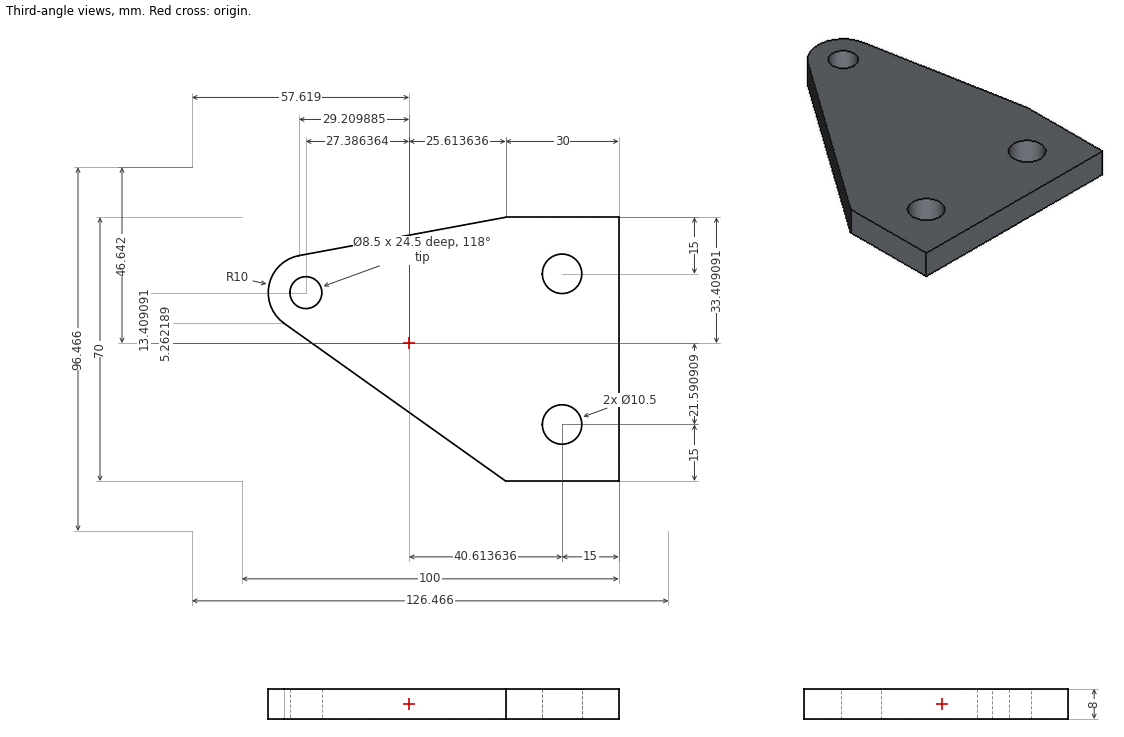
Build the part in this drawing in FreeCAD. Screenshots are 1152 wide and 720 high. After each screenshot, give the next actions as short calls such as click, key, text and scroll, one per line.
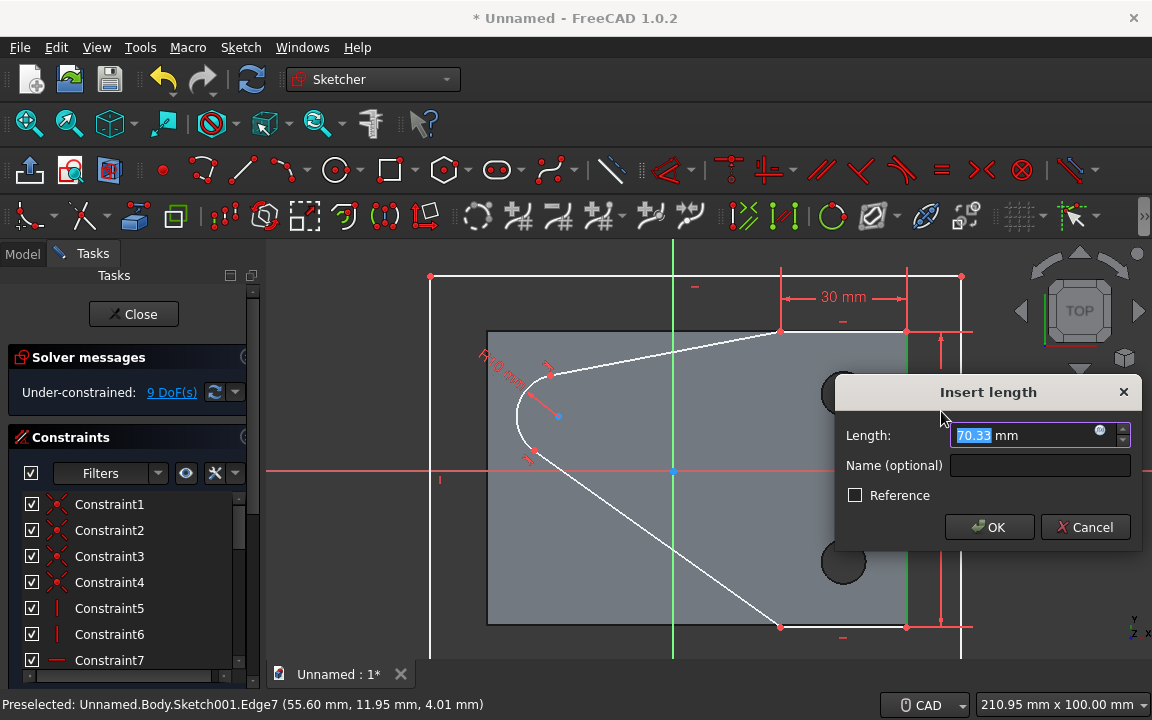
text(70)
key(Return)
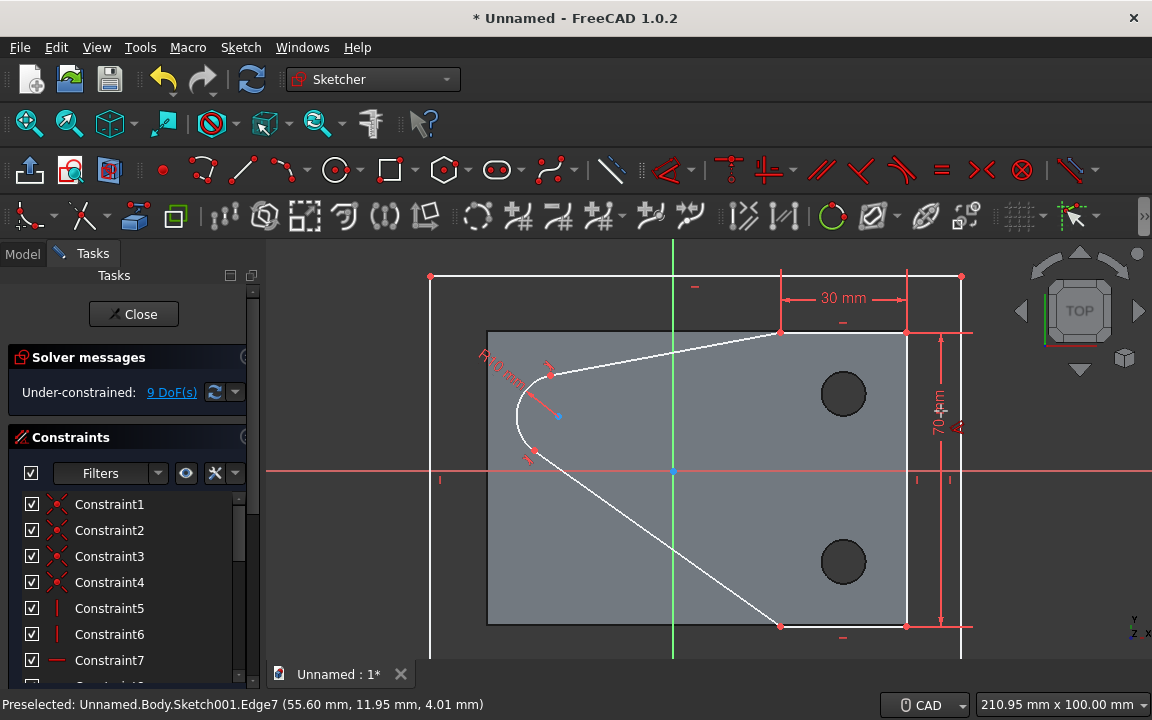
click(869, 627)
click(844, 593)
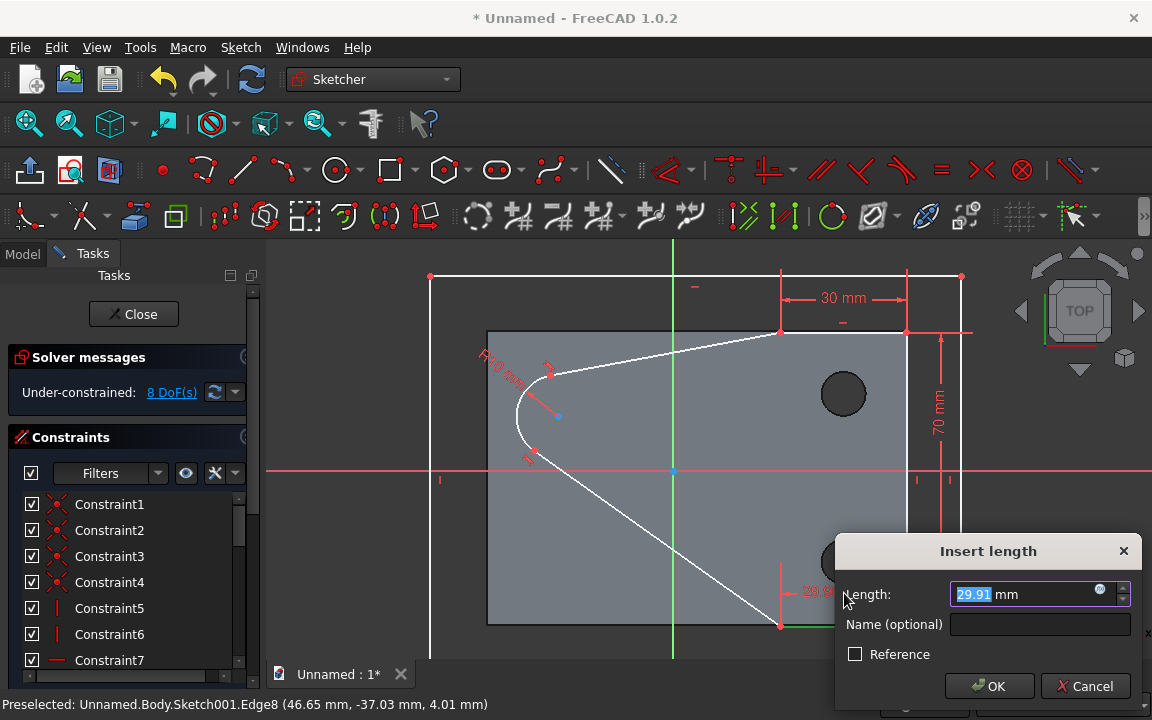
text(30)
key(Return)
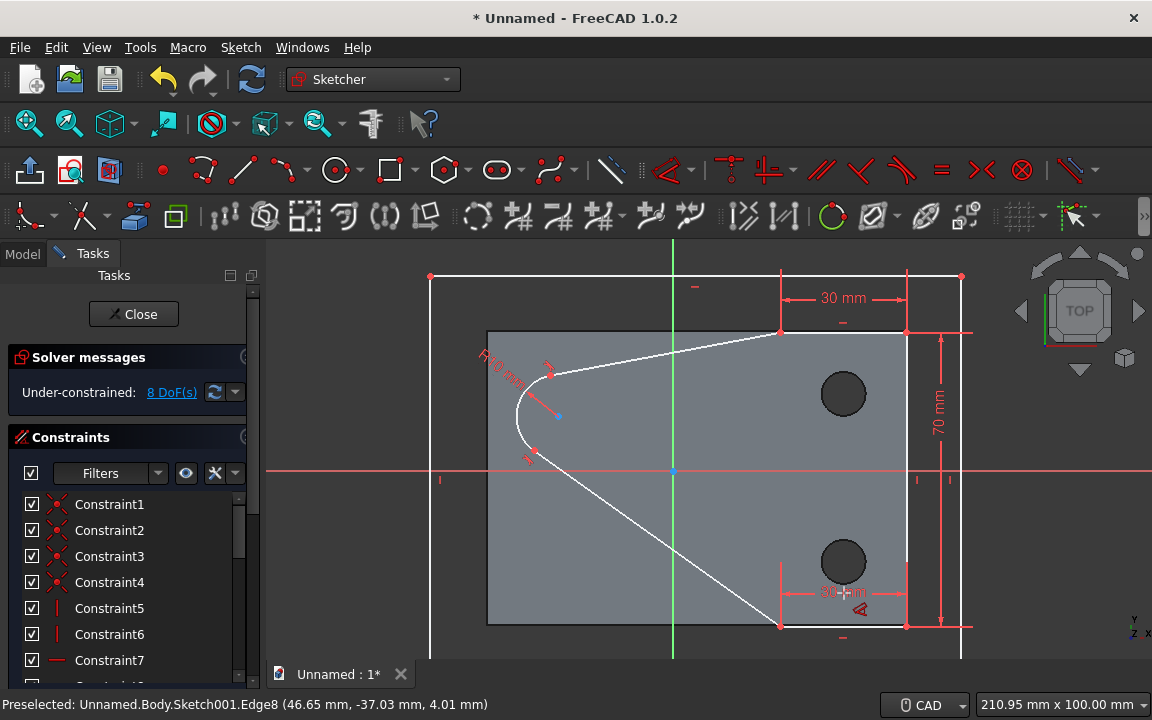
click(430, 398)
click(396, 454)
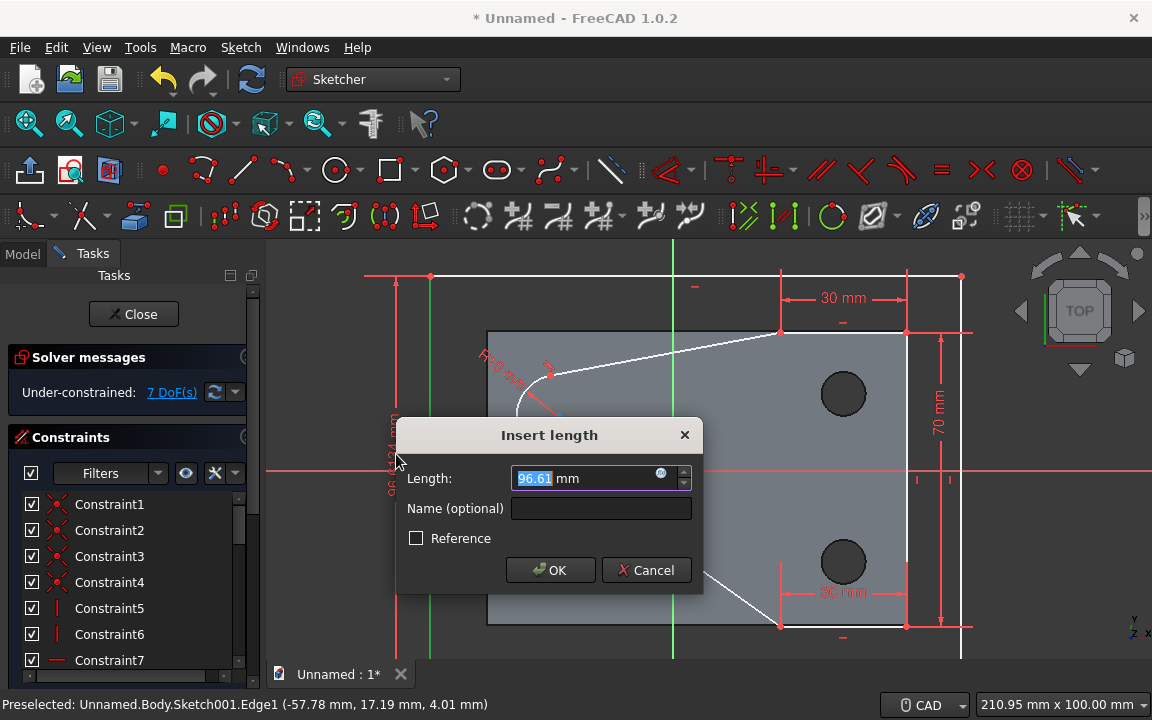
text(96.466)
key(Return)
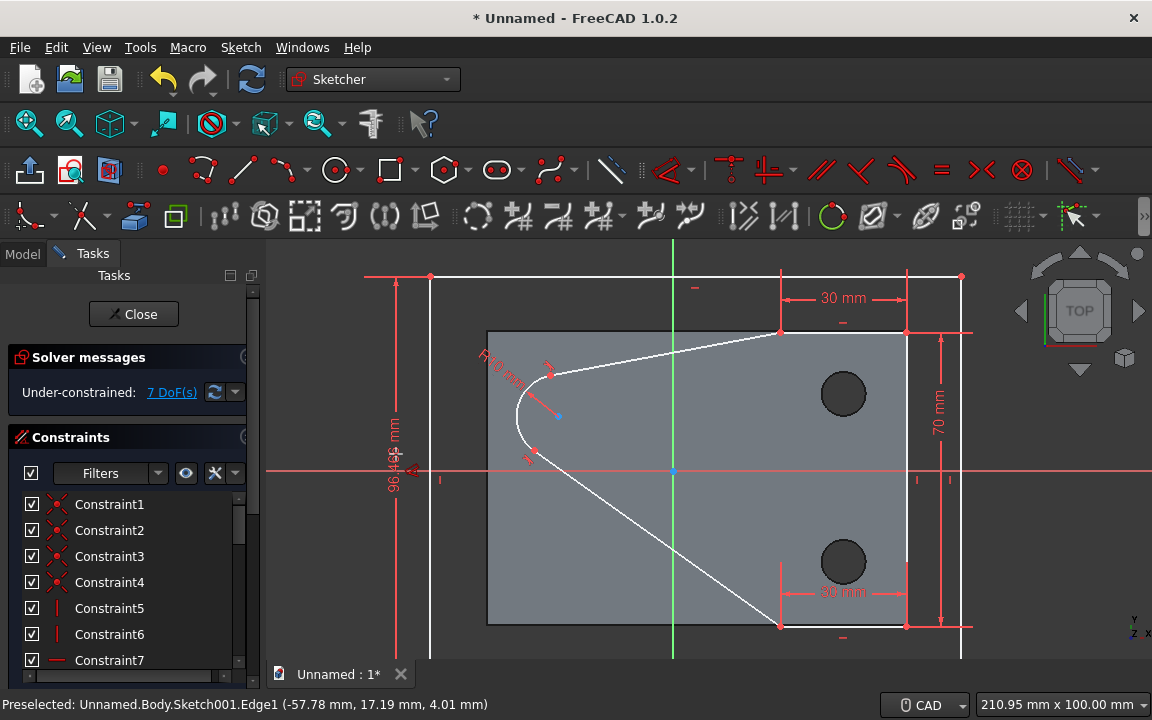
scroll(526, 390, down, 2)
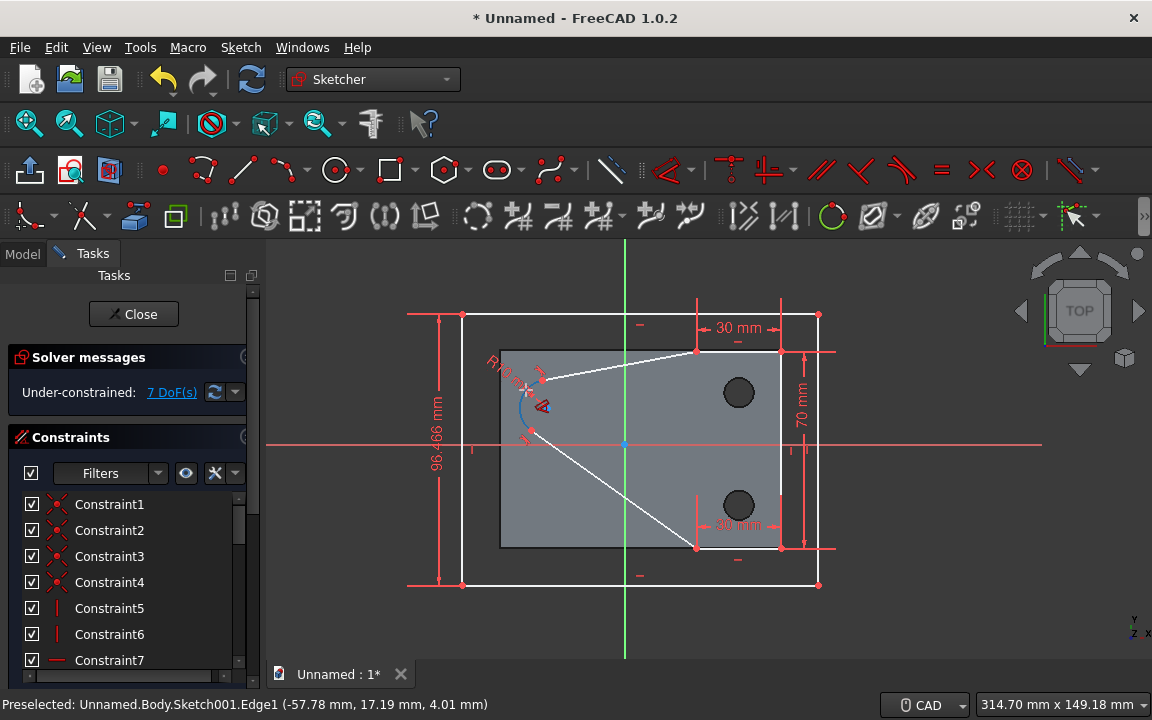
click(569, 586)
click(640, 620)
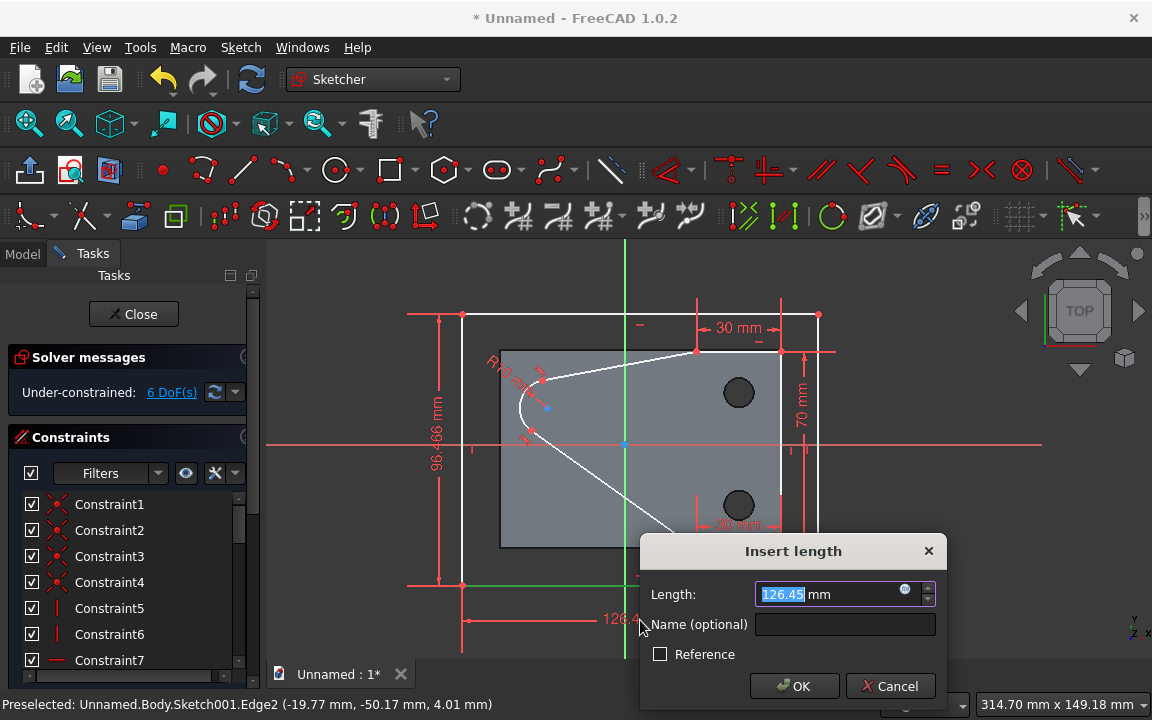
text(126.466)
key(Return)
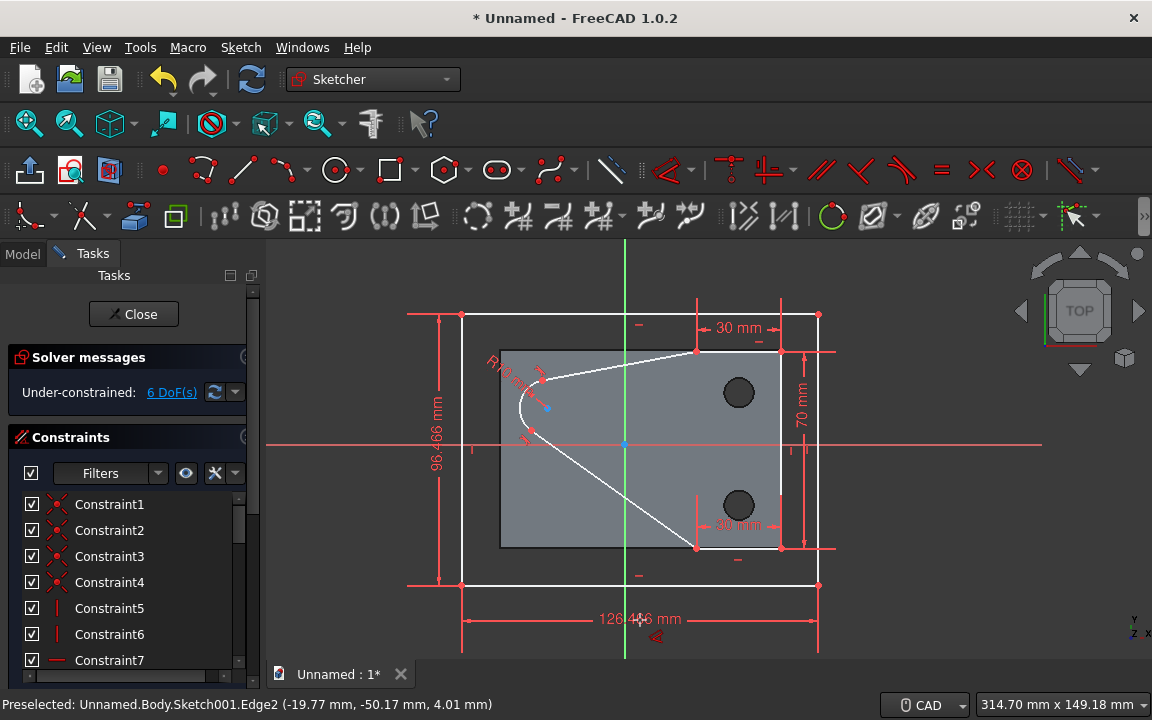
click(462, 314)
click(543, 280)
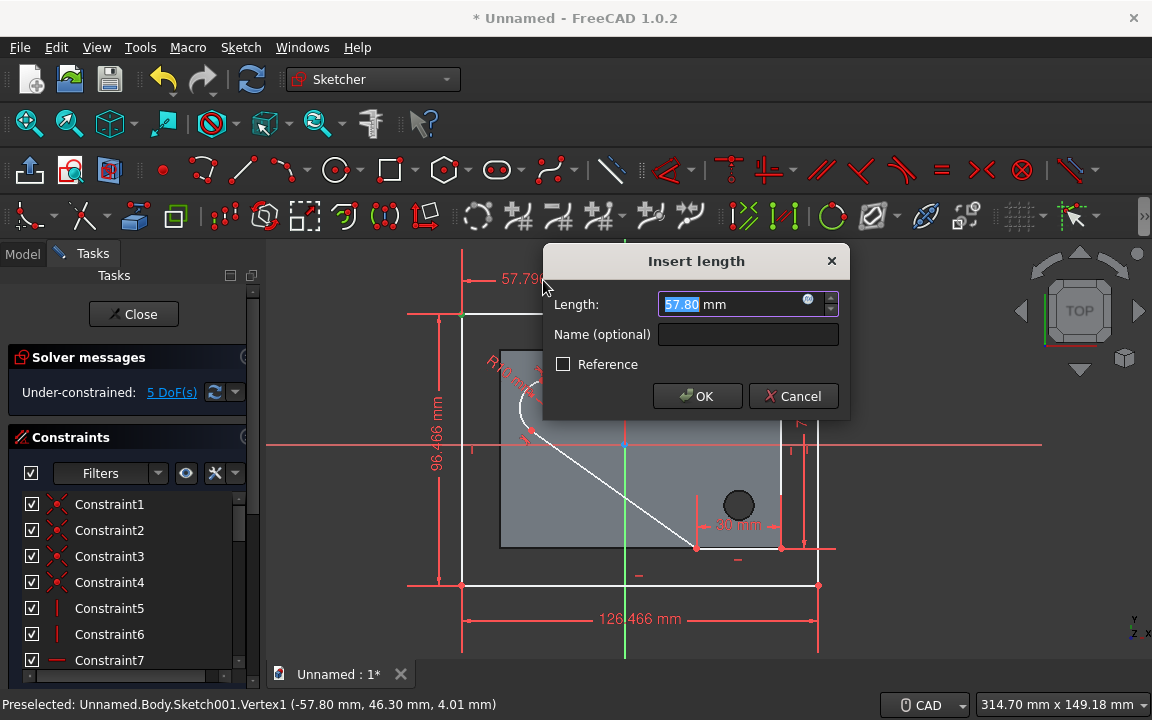
text(57.619)
key(Return)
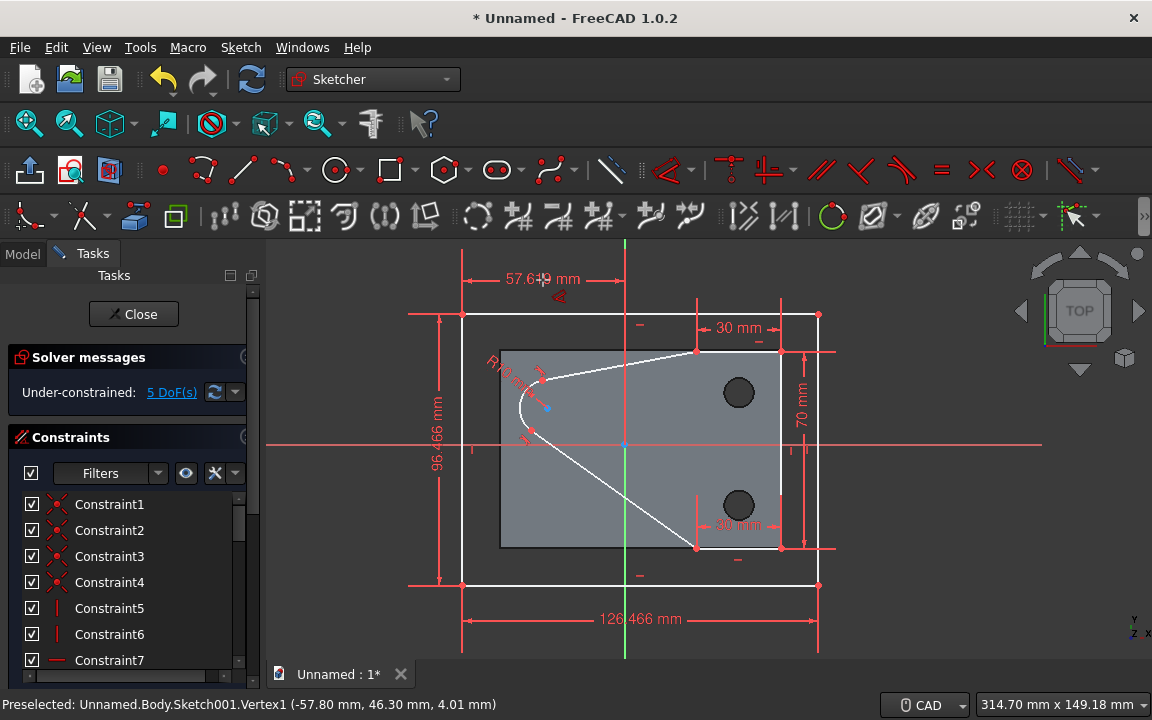
click(462, 314)
click(428, 379)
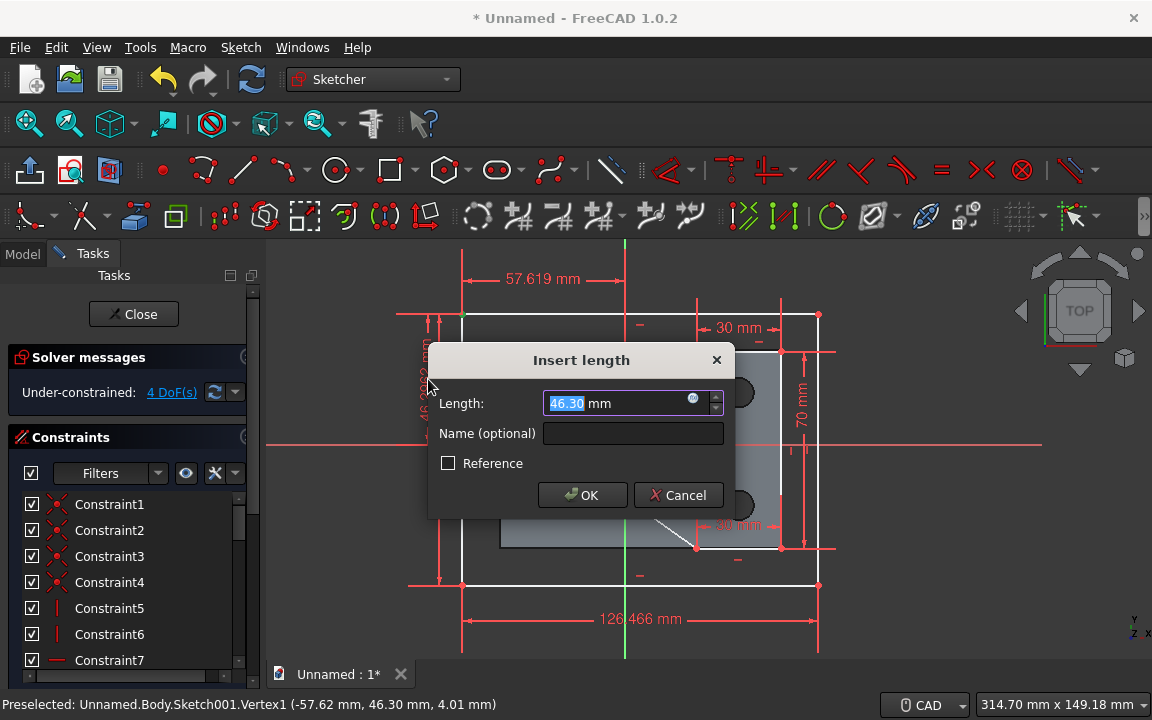
text(46.642)
key(Return)